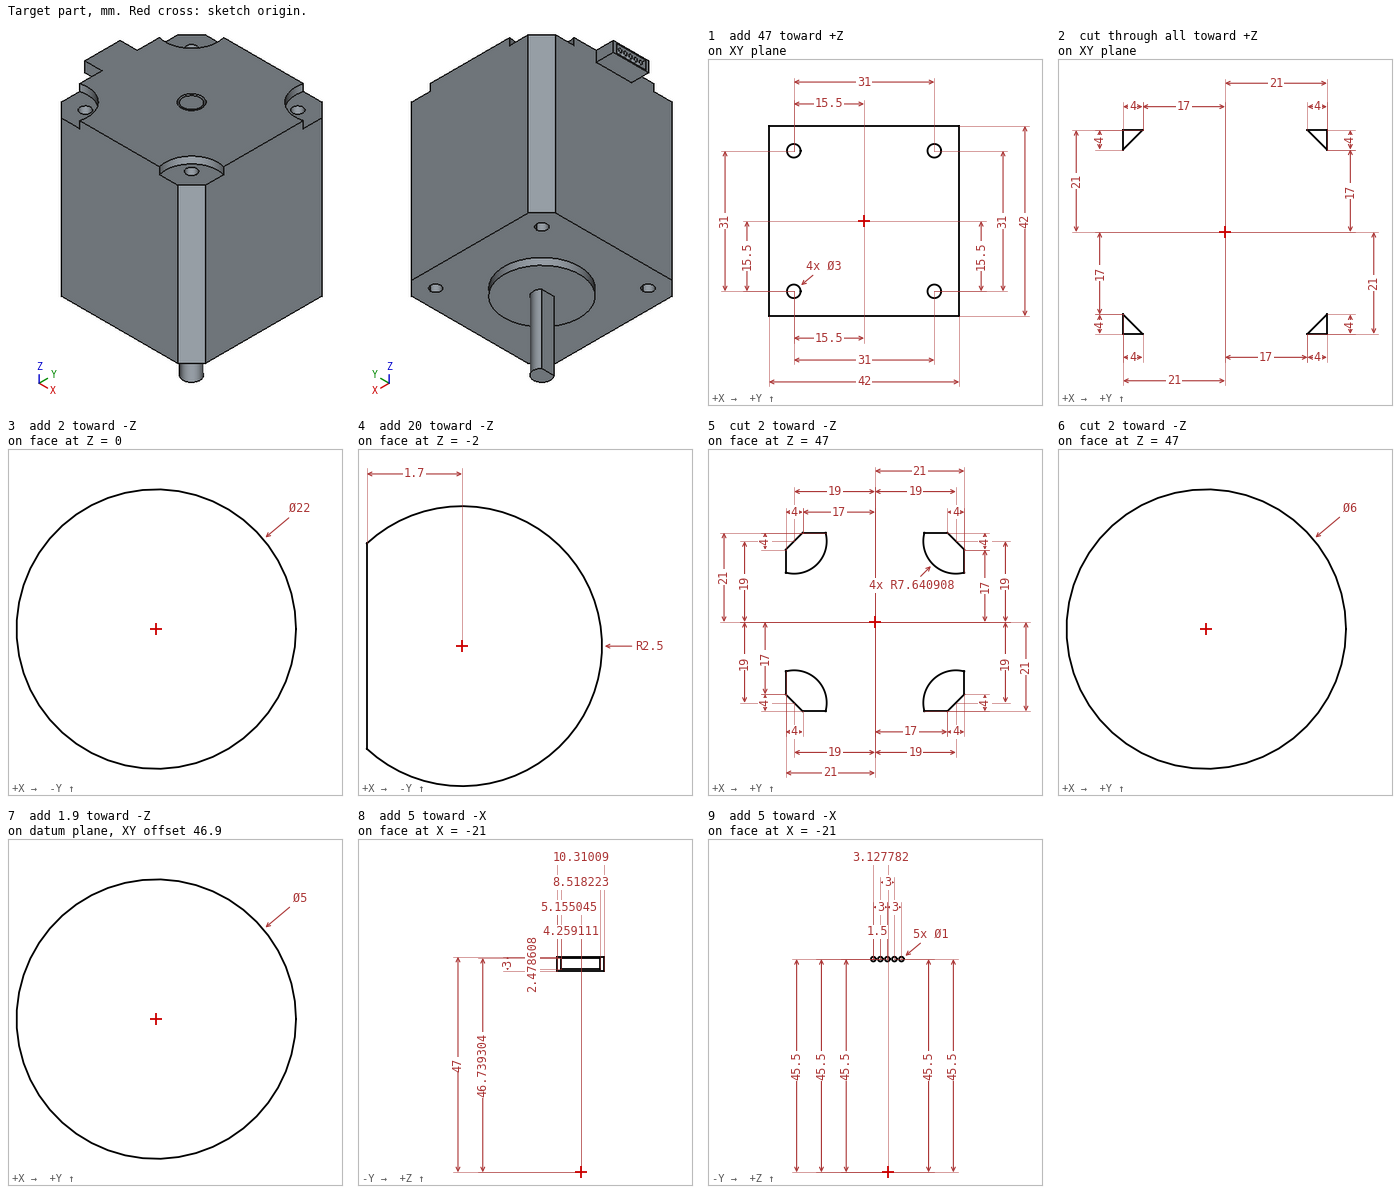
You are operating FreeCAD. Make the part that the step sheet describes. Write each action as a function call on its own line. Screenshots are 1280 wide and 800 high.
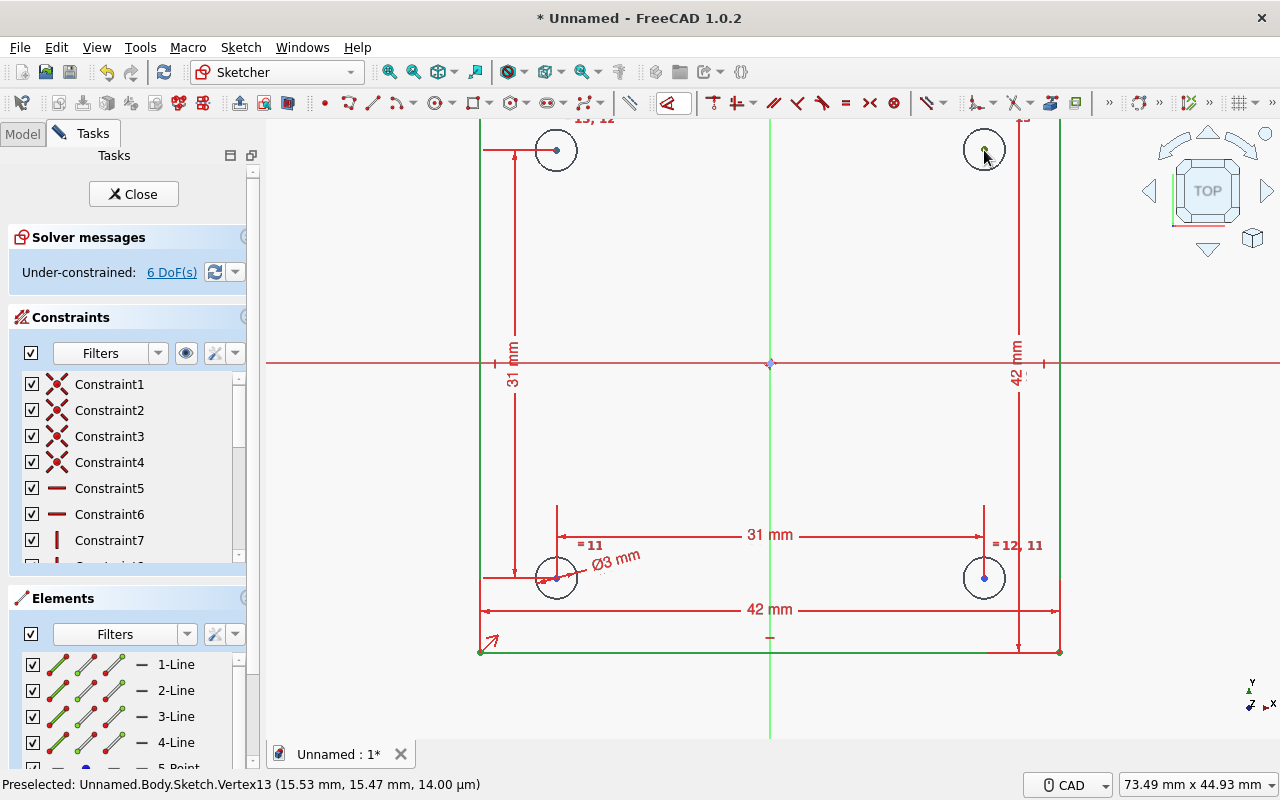
key(l)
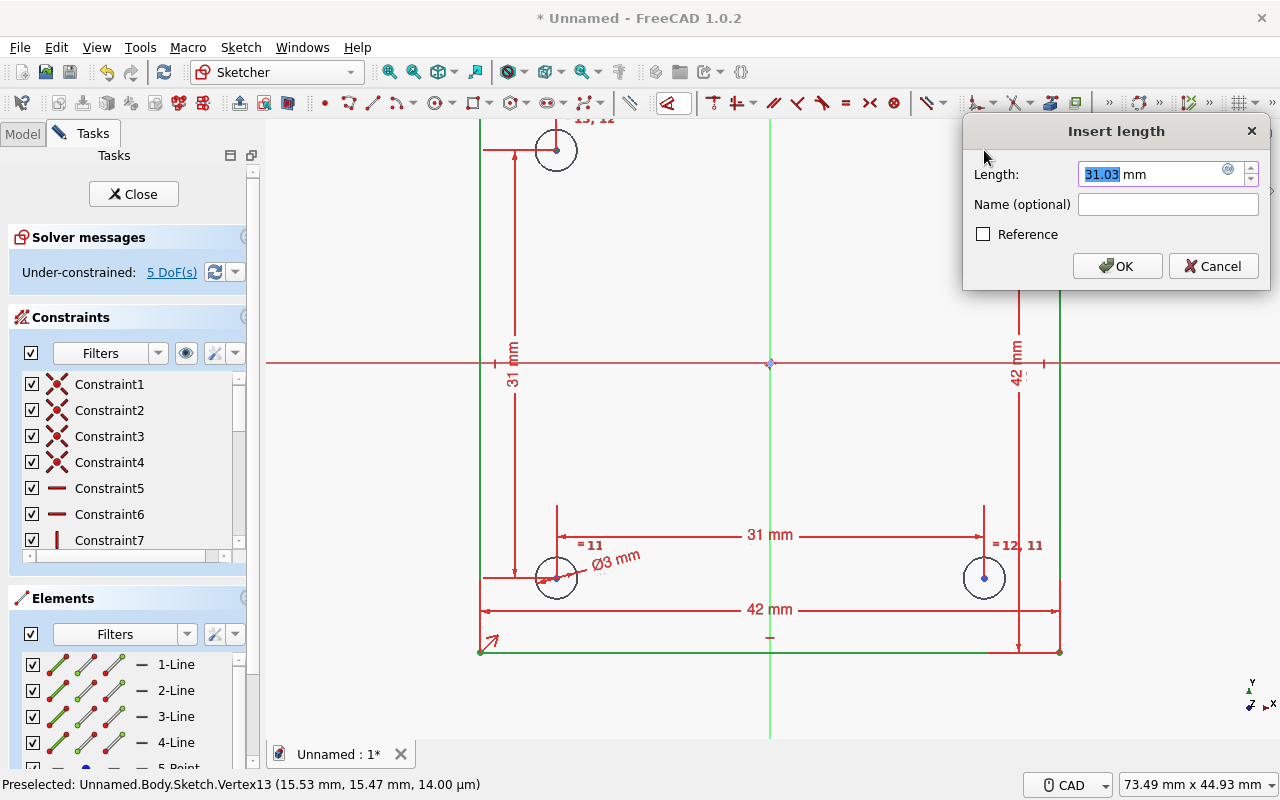
text(31)
key(Return)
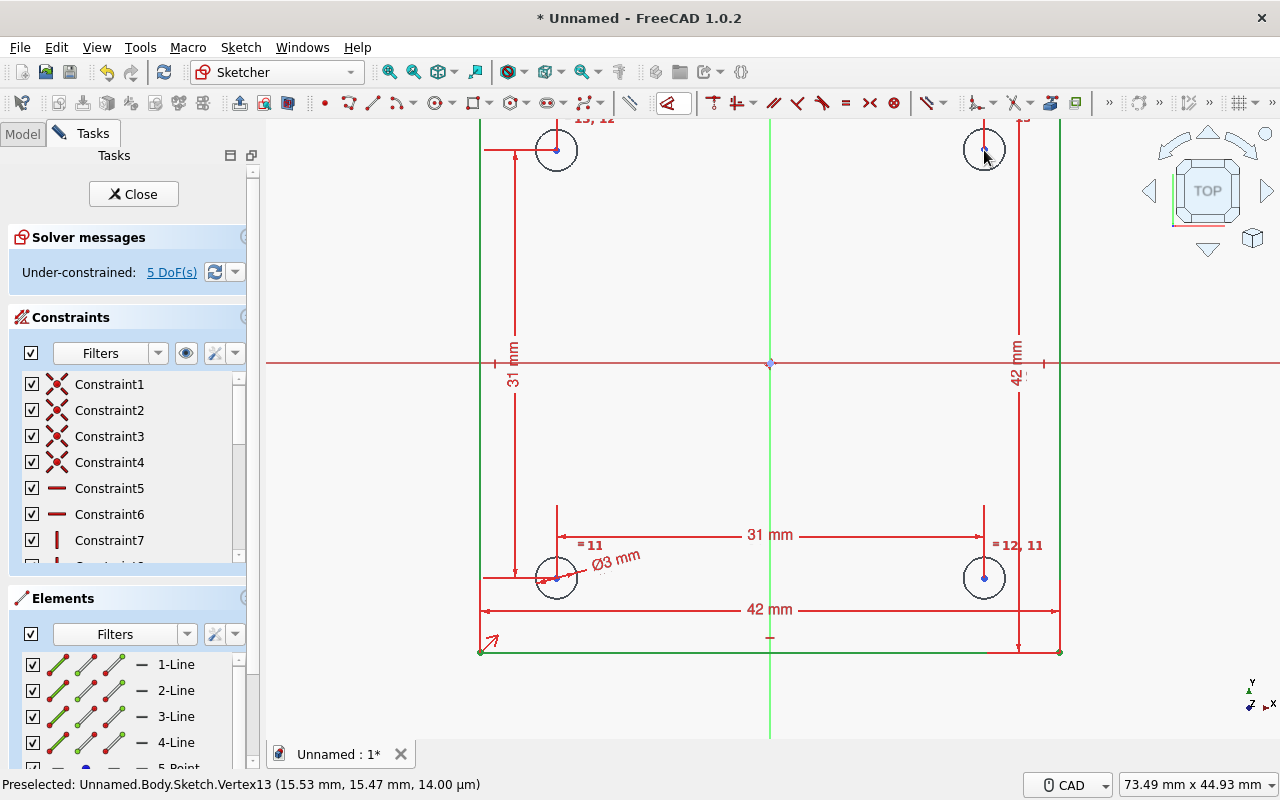
click(984, 578)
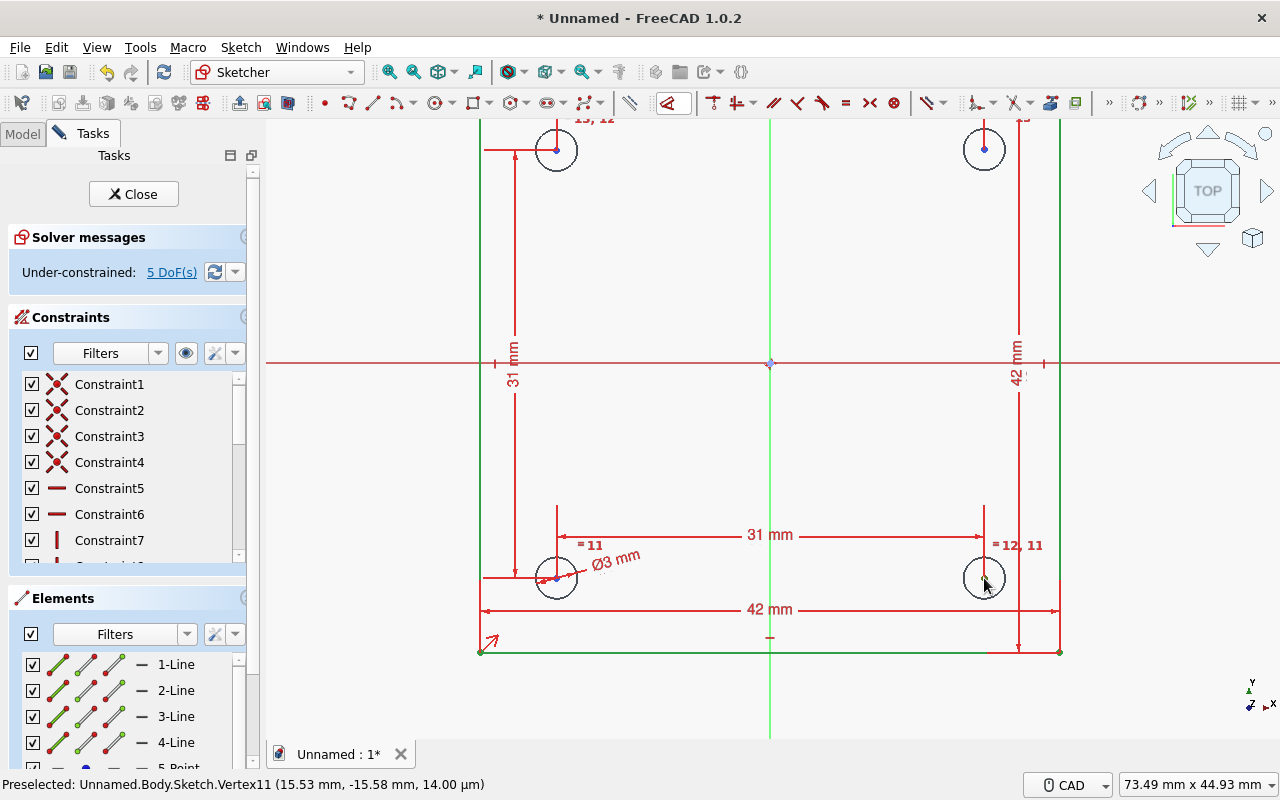
click(984, 150)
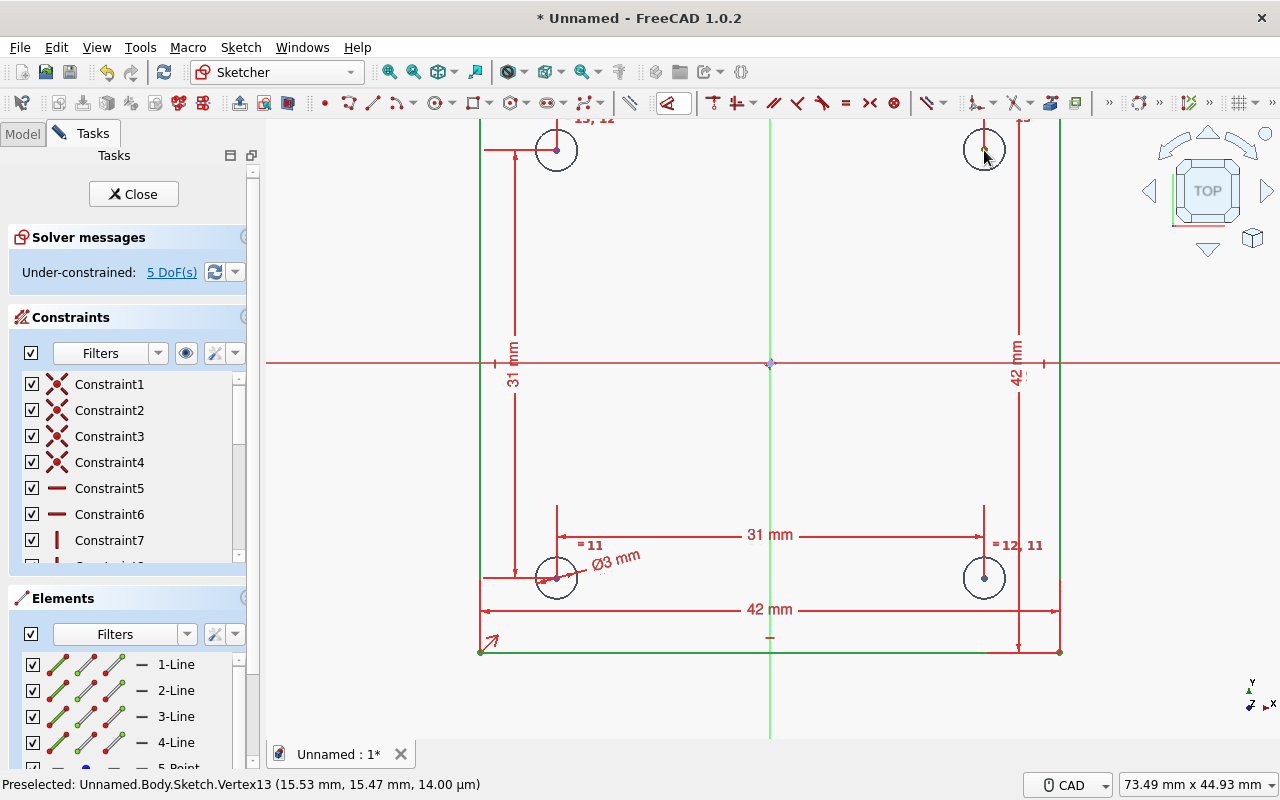
key(i)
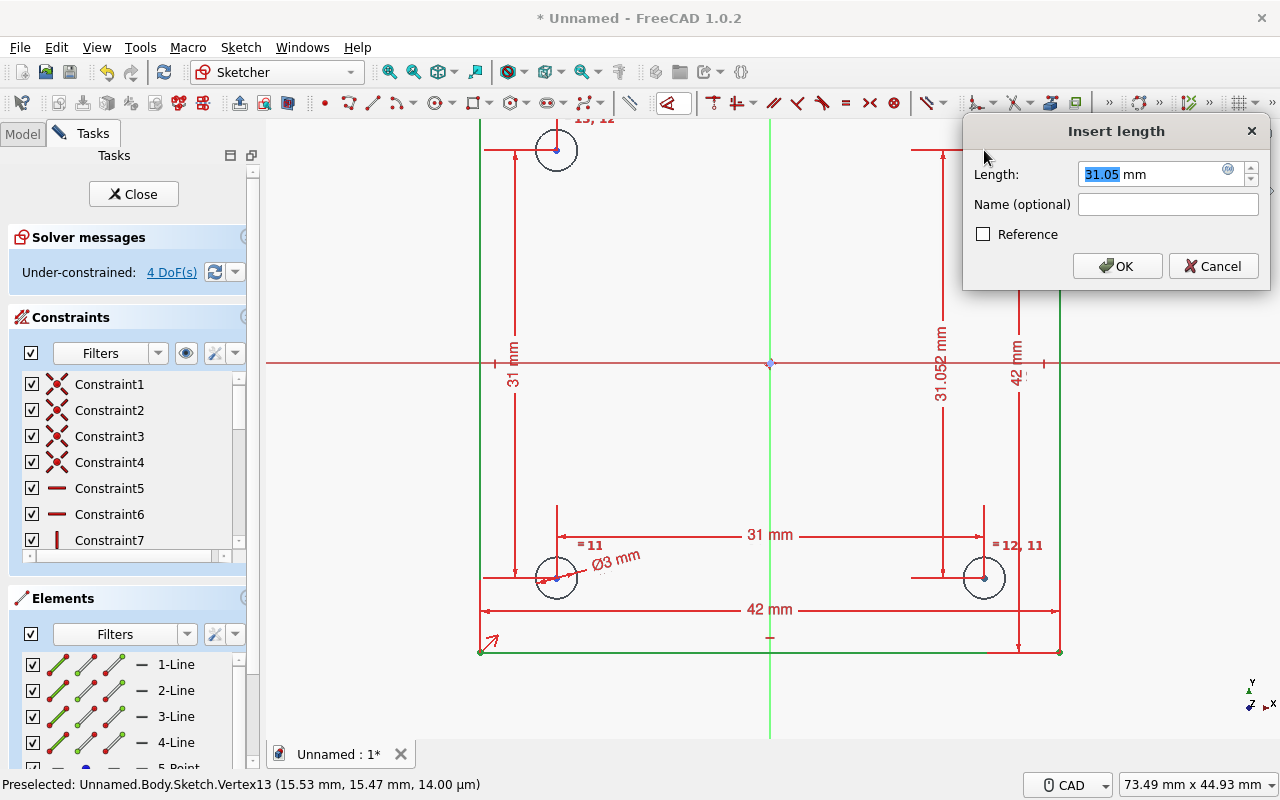
text(31)
key(Return)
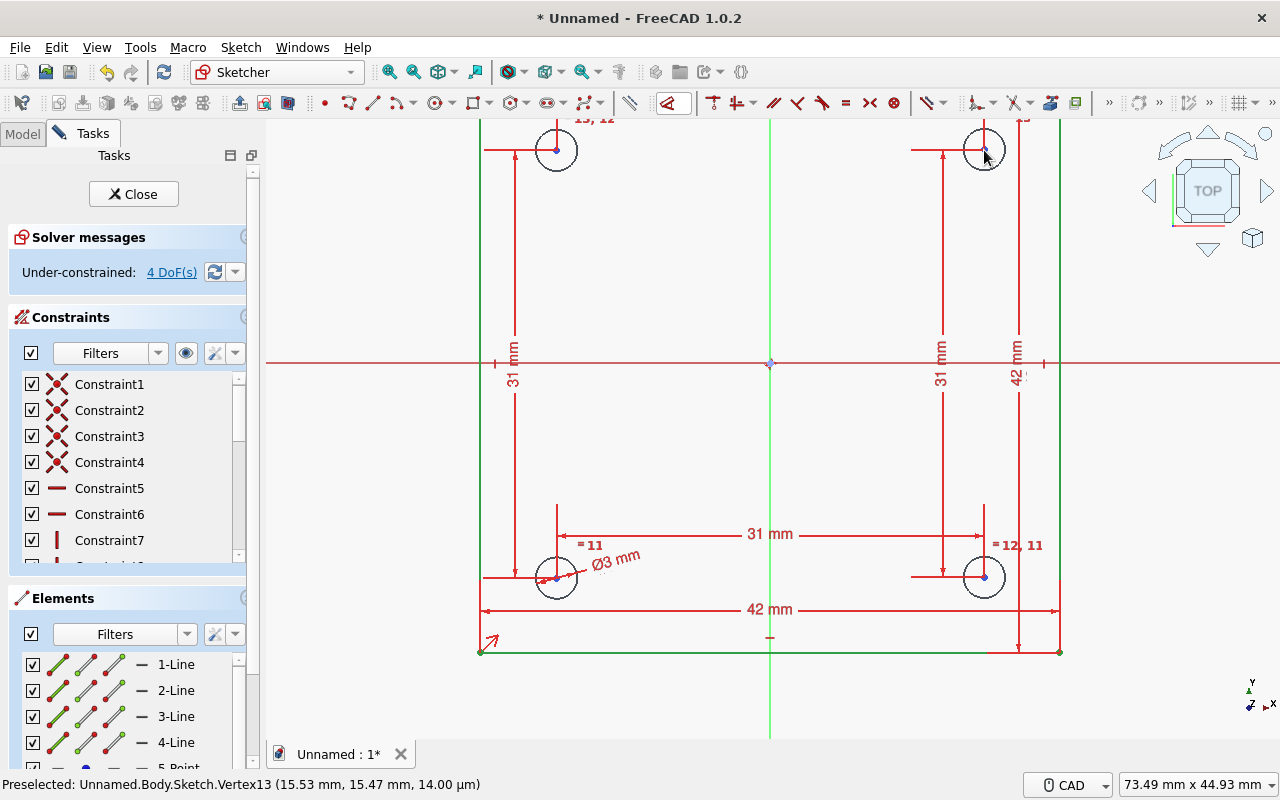
click(557, 578)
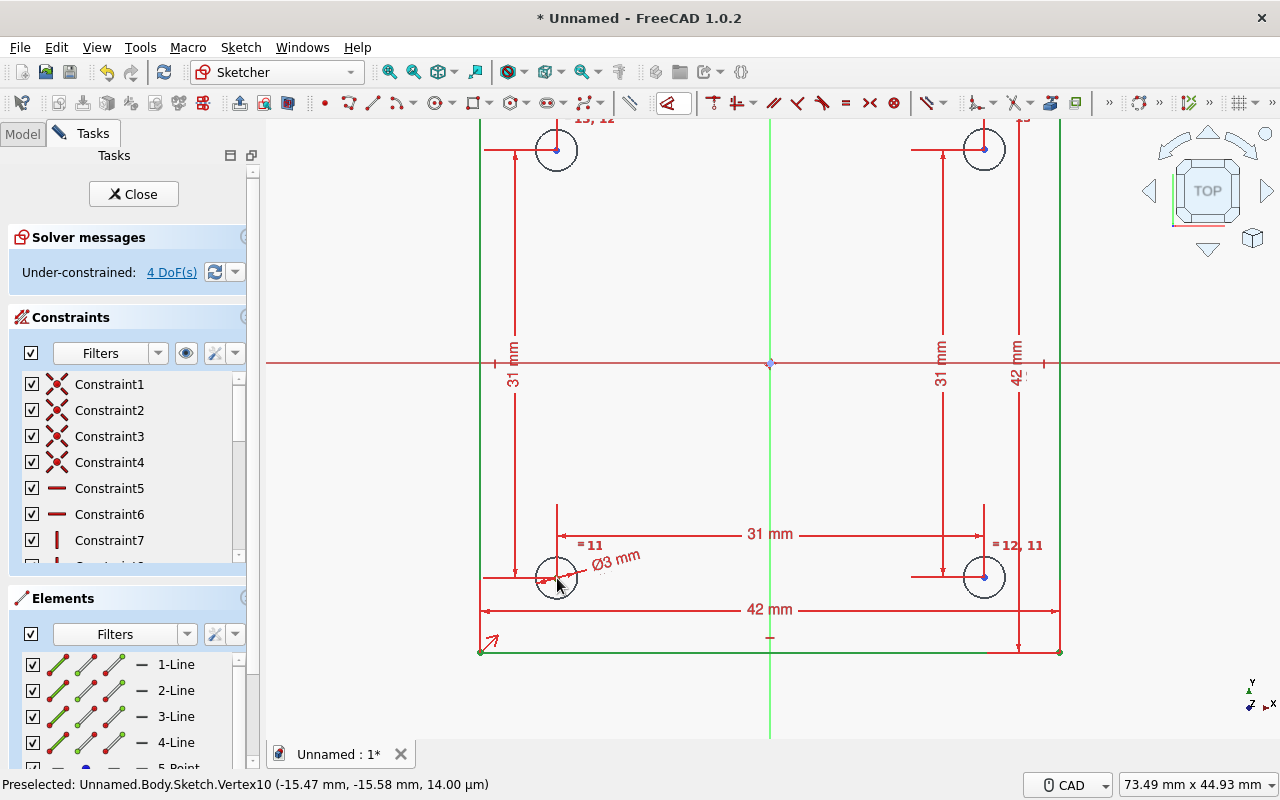
click(686, 104)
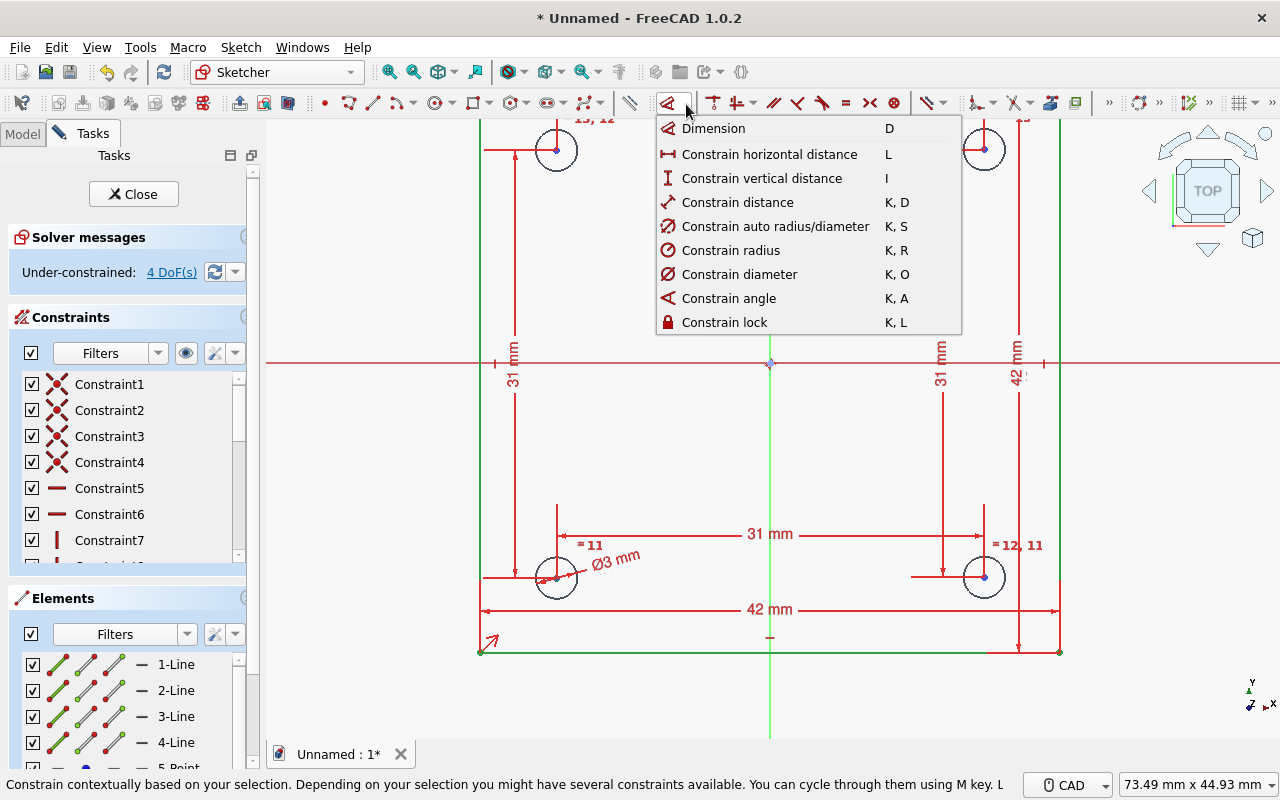
click(809, 154)